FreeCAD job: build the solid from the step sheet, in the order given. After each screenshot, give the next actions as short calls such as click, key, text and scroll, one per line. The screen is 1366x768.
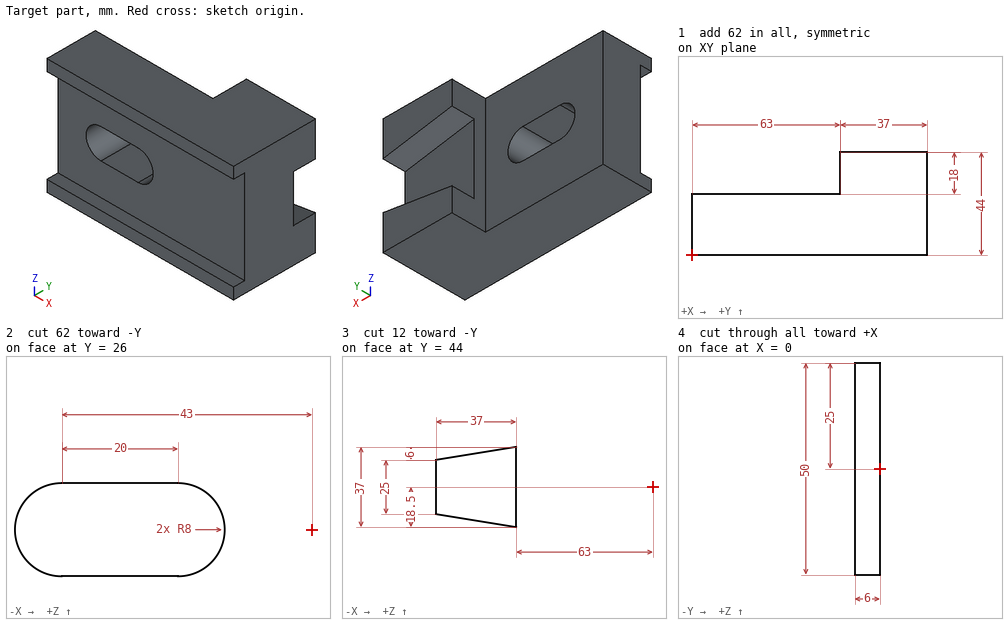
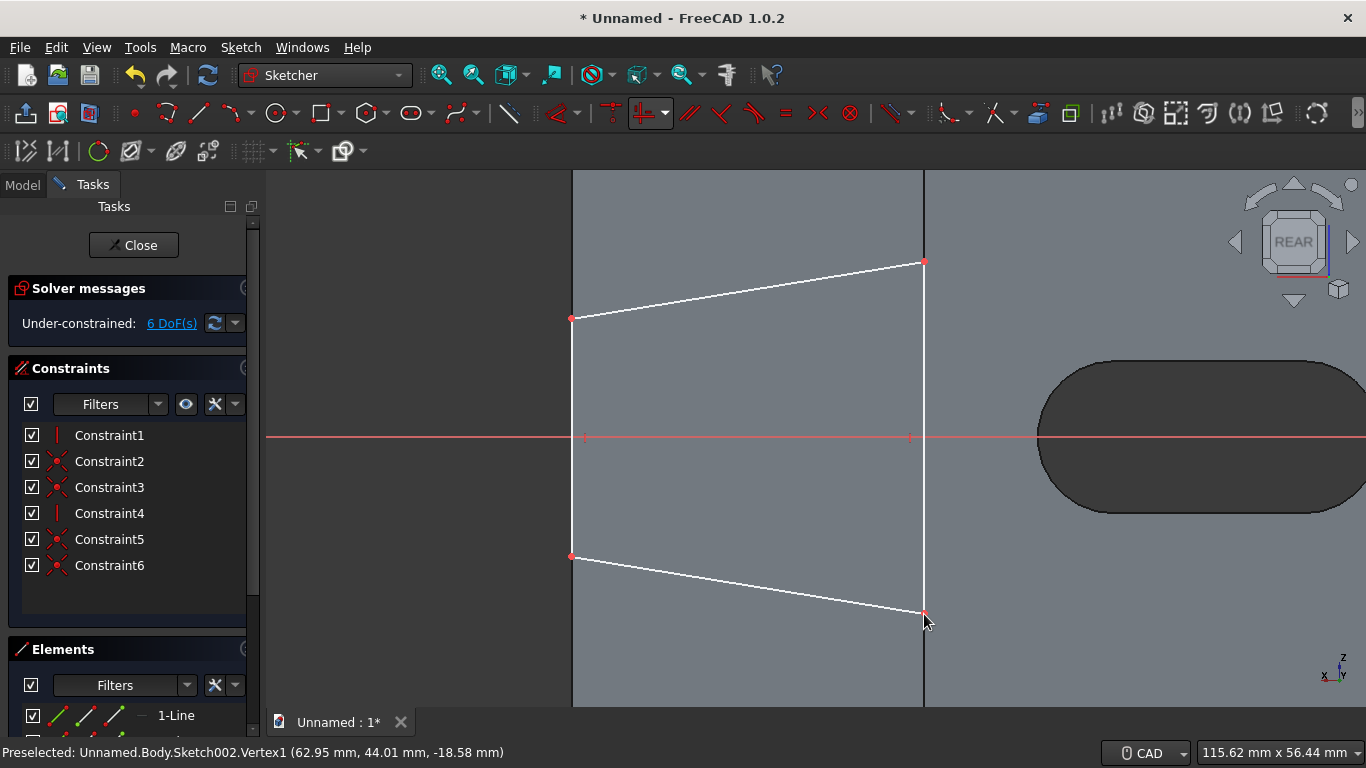
click(556, 114)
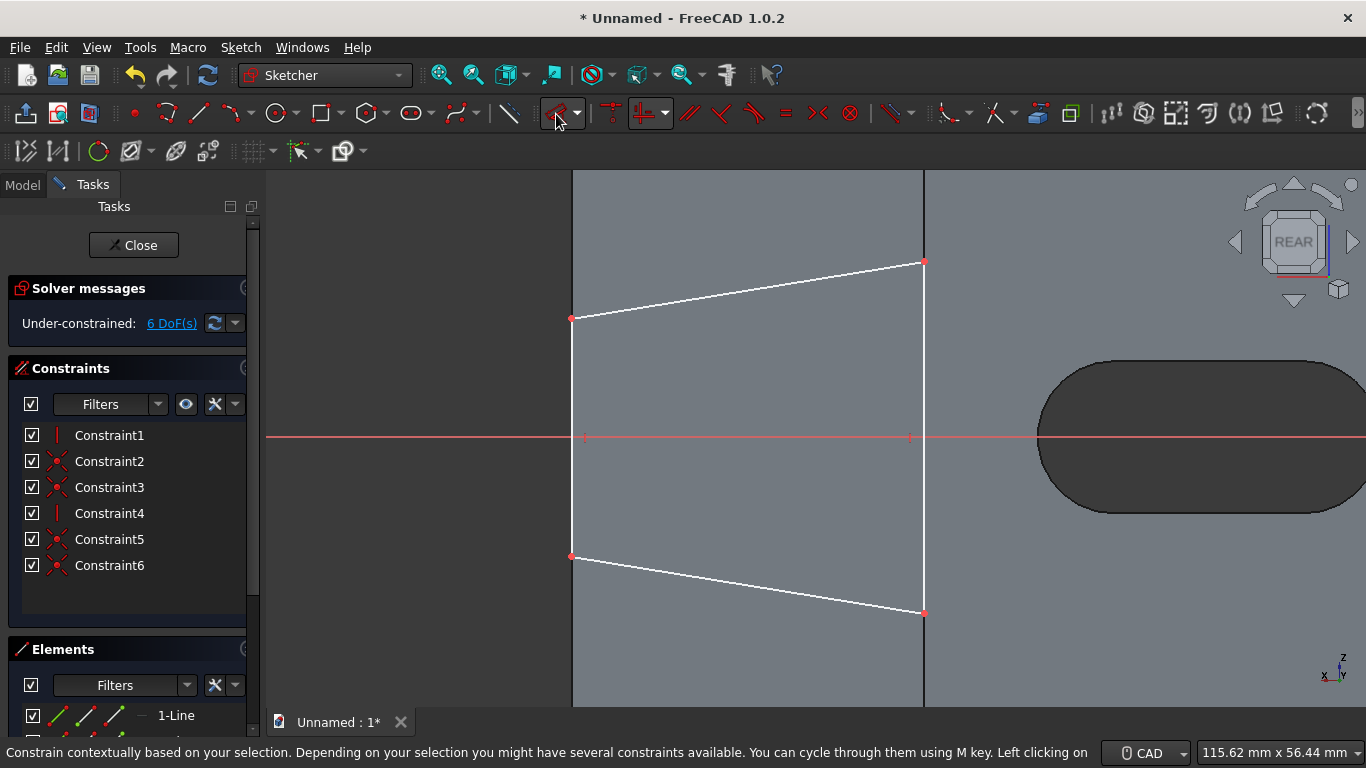
click(924, 508)
click(958, 357)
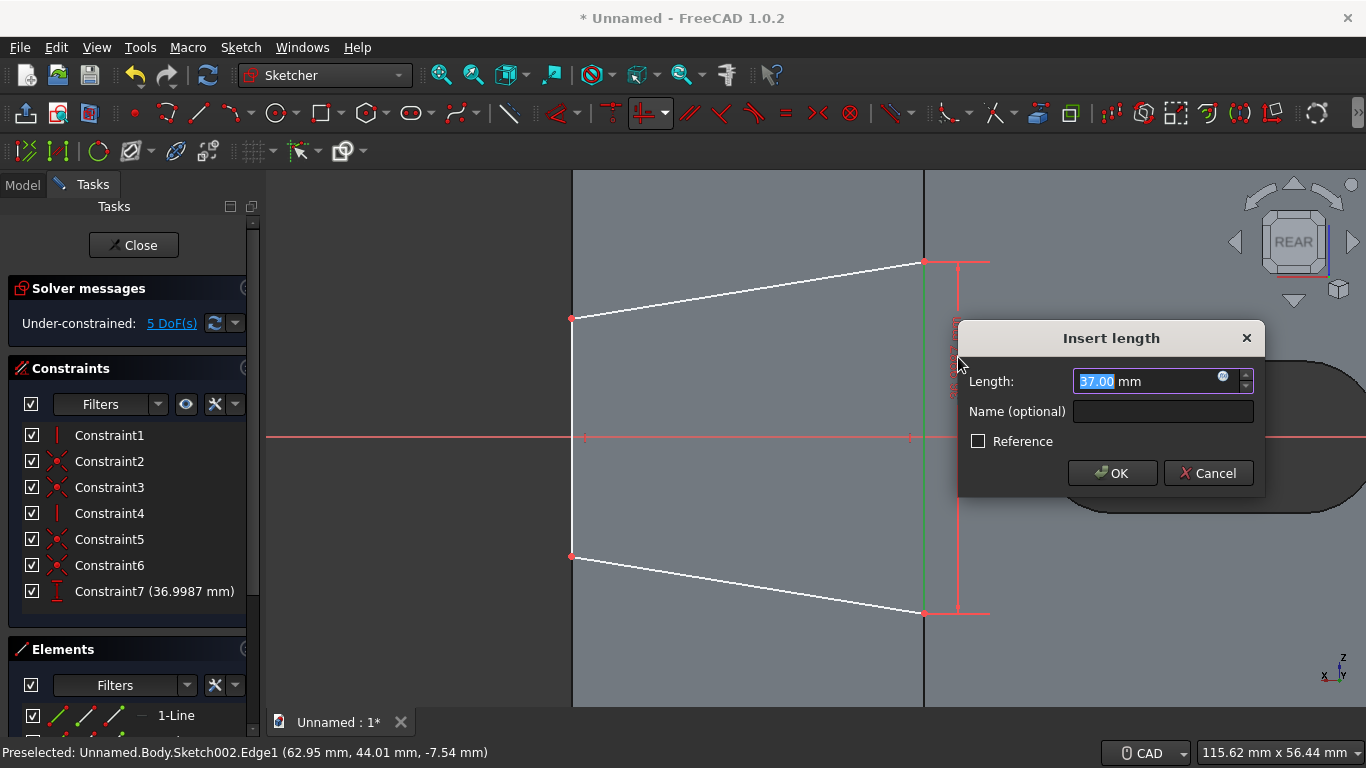
text(37)
key(Return)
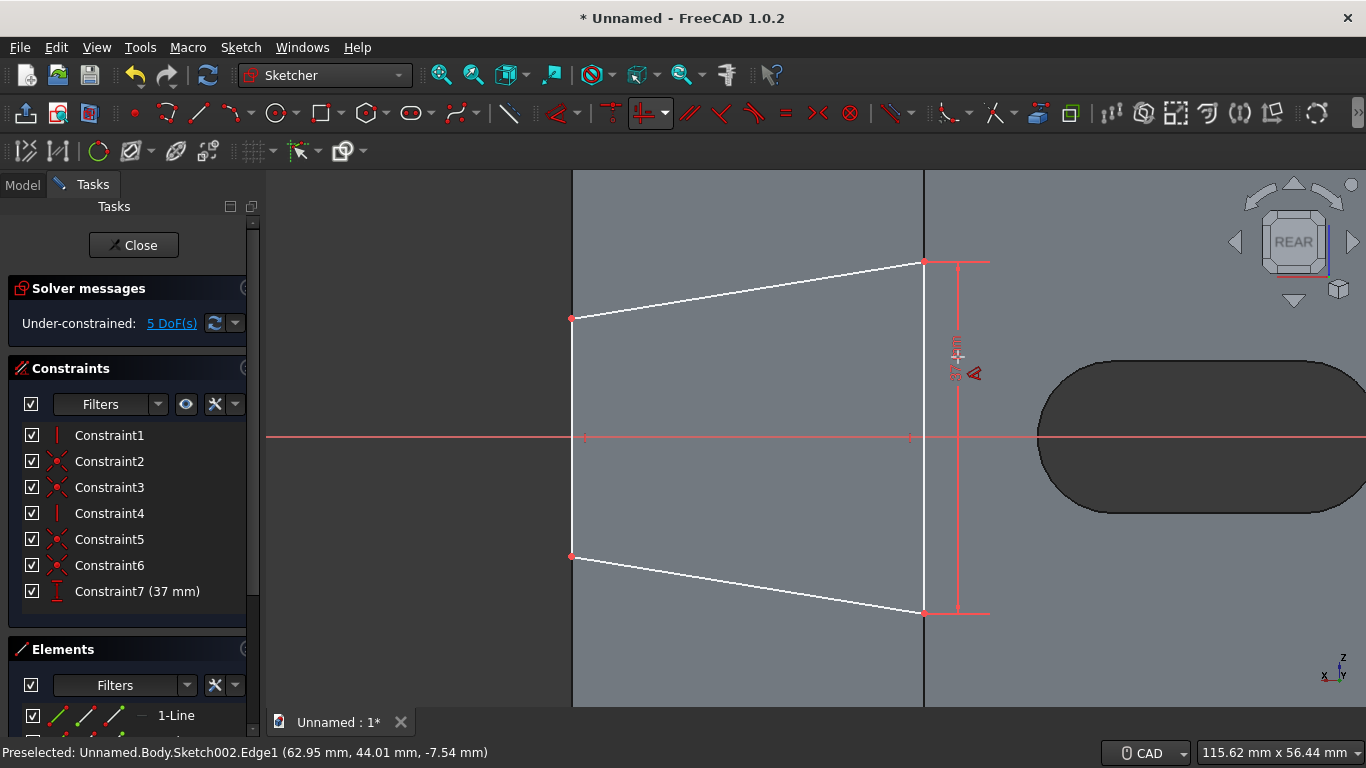
click(572, 390)
click(538, 383)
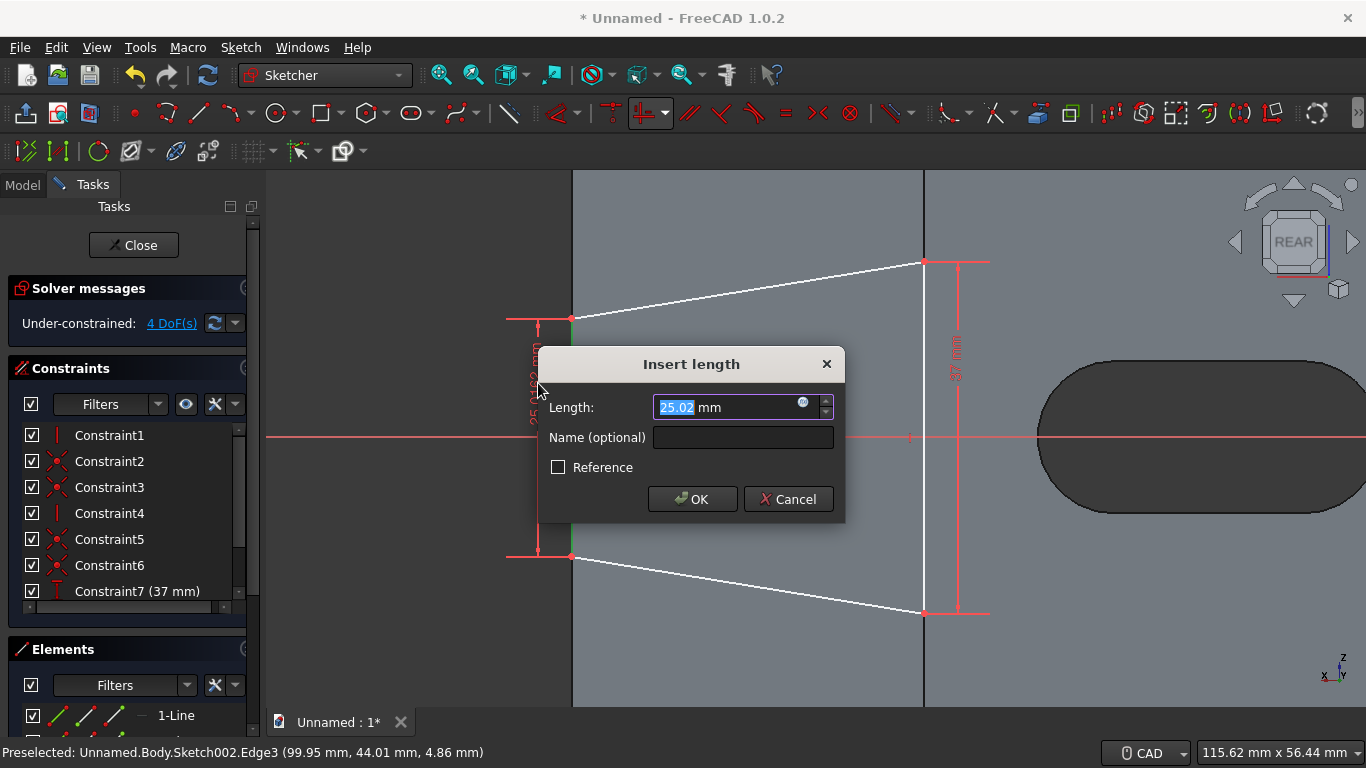
text(25)
key(Return)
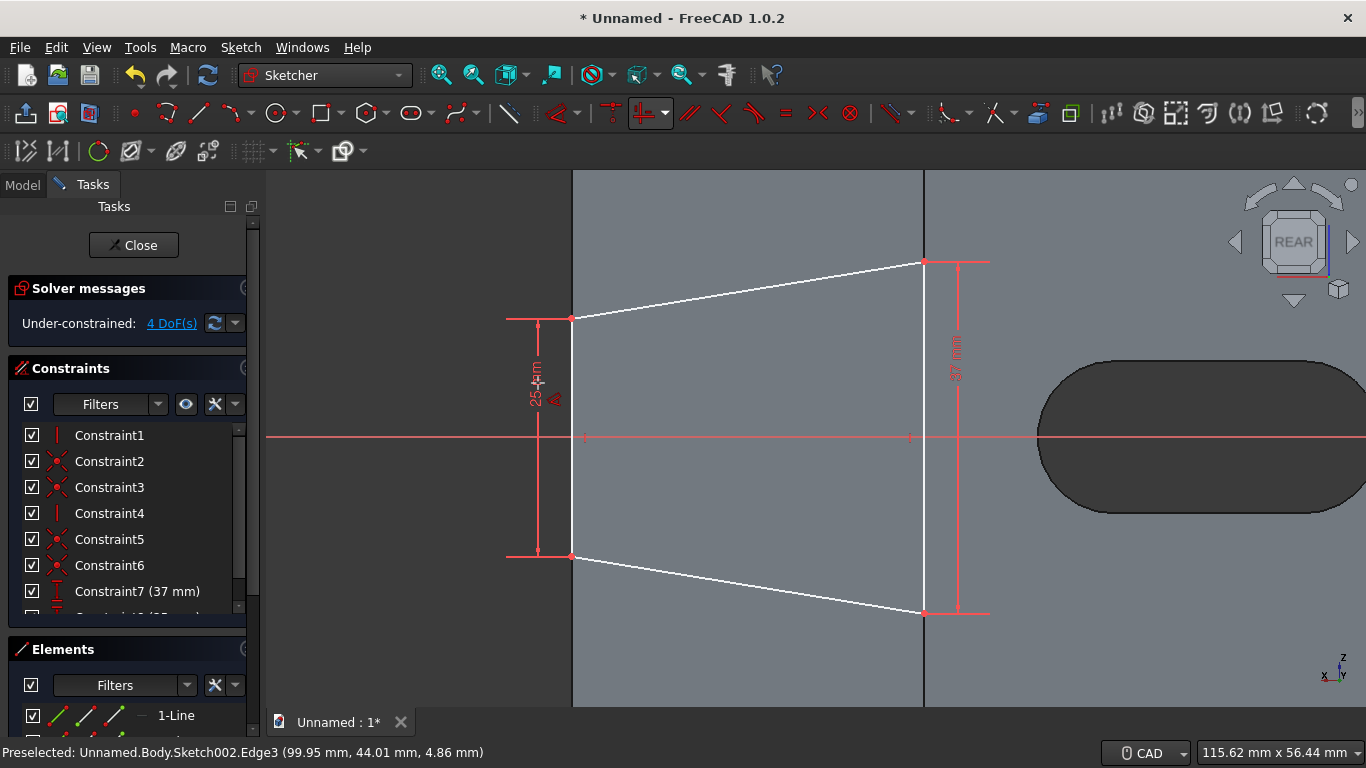
click(818, 279)
click(958, 290)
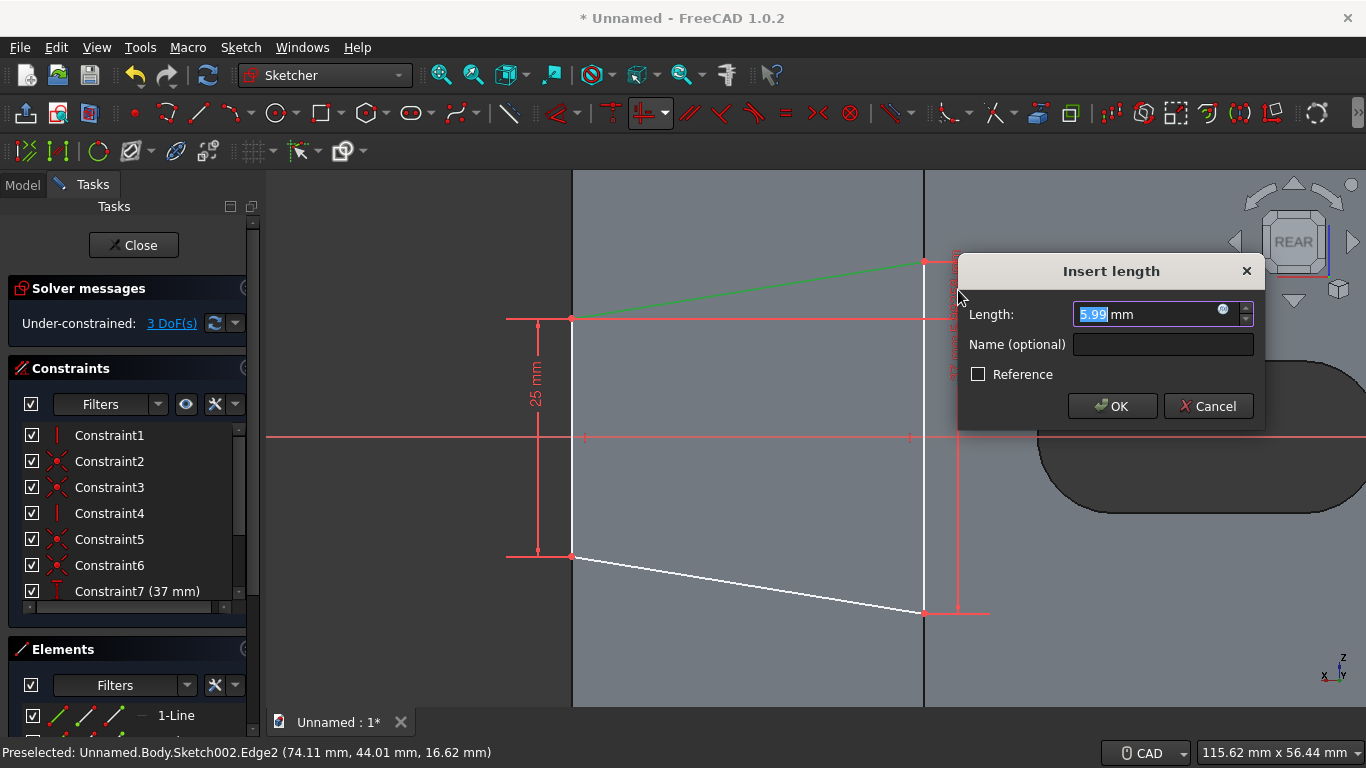
text(6)
key(Return)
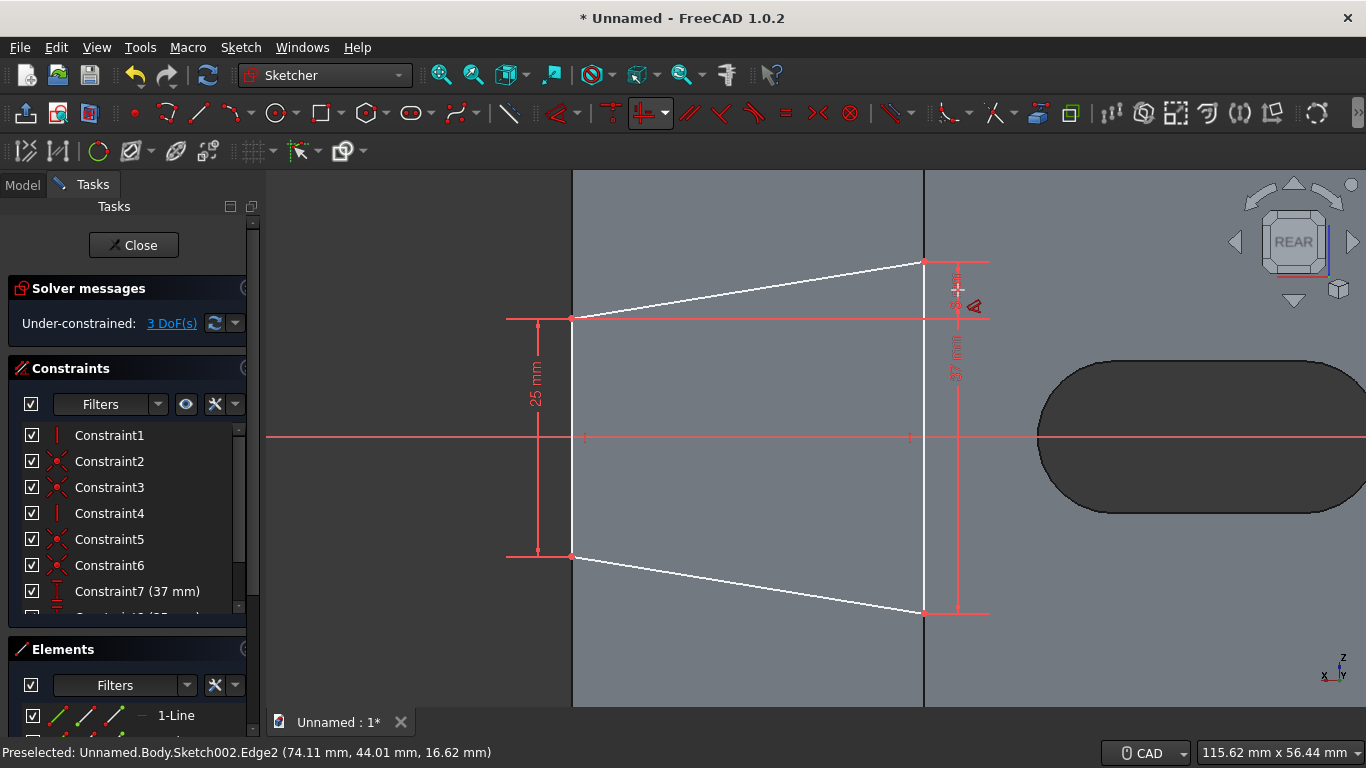
click(924, 614)
click(1063, 648)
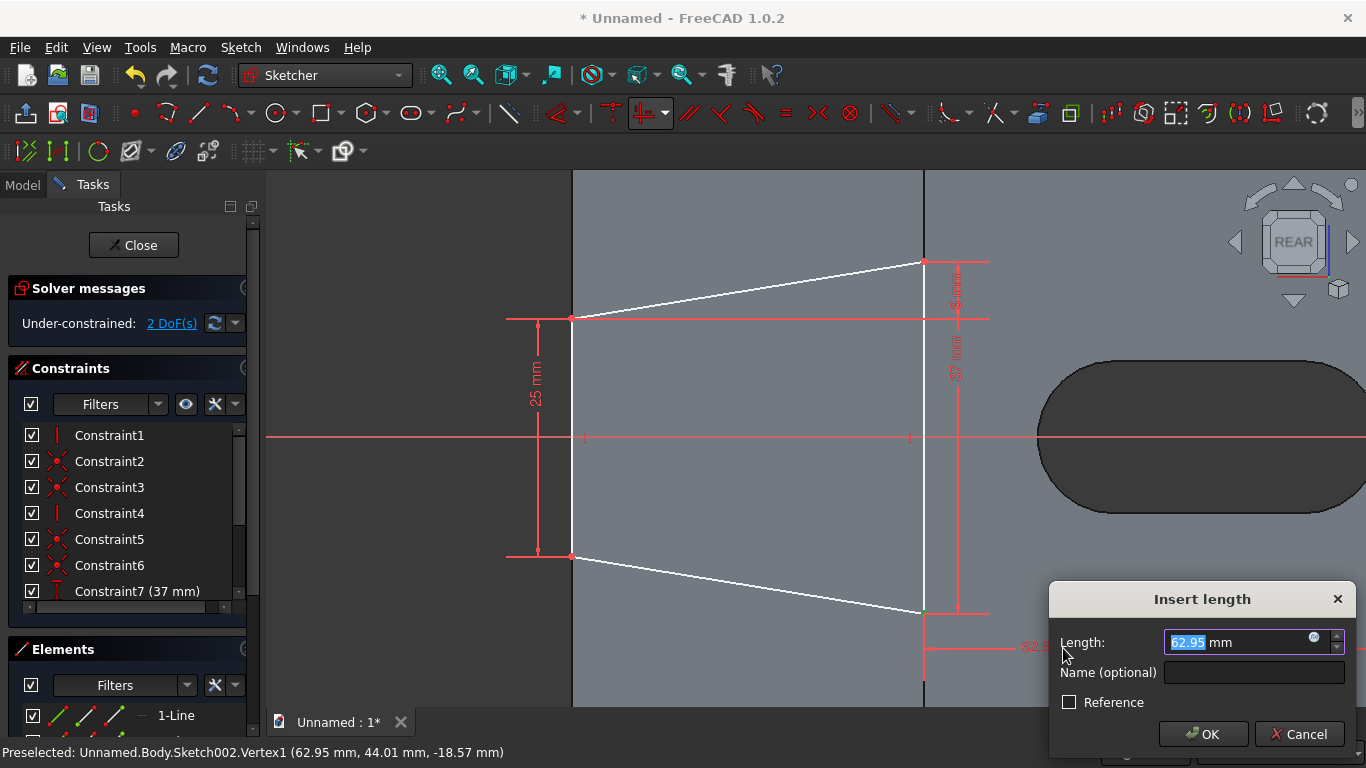
text(63)
key(Return)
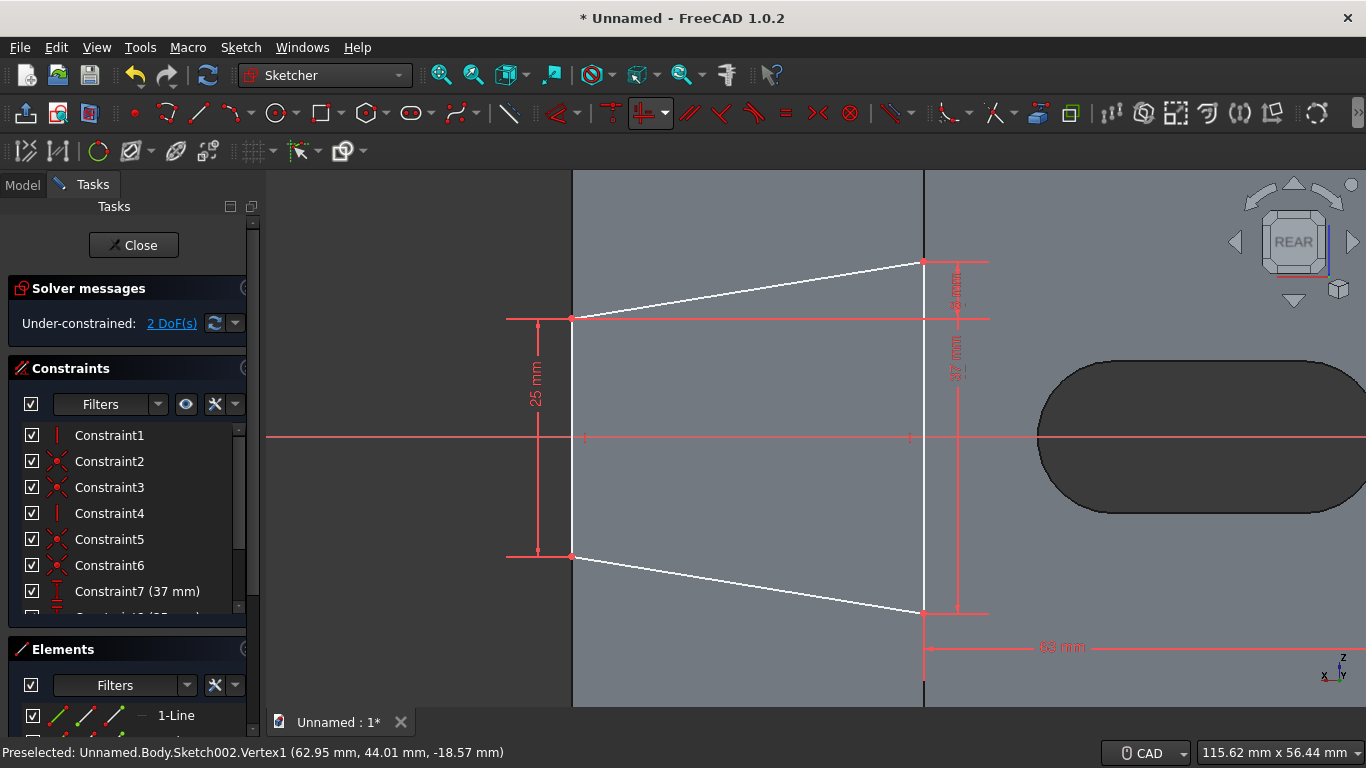
click(818, 279)
click(748, 228)